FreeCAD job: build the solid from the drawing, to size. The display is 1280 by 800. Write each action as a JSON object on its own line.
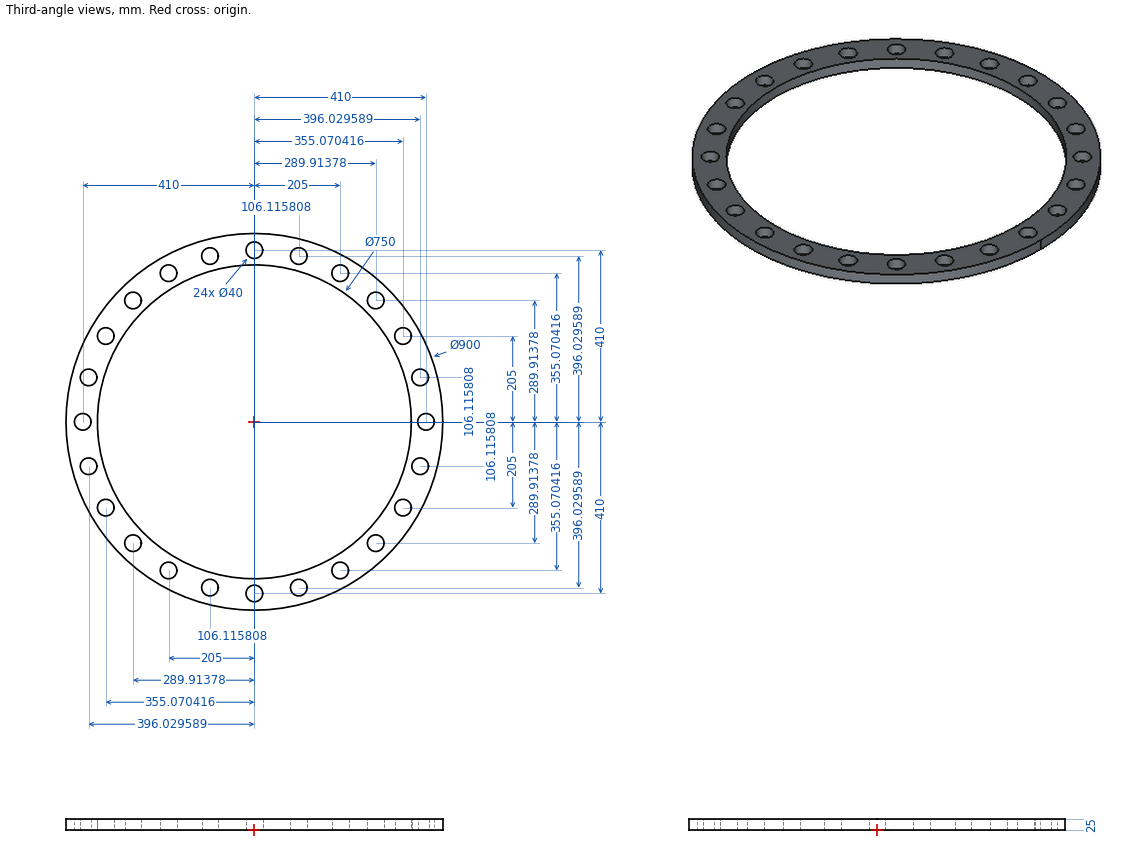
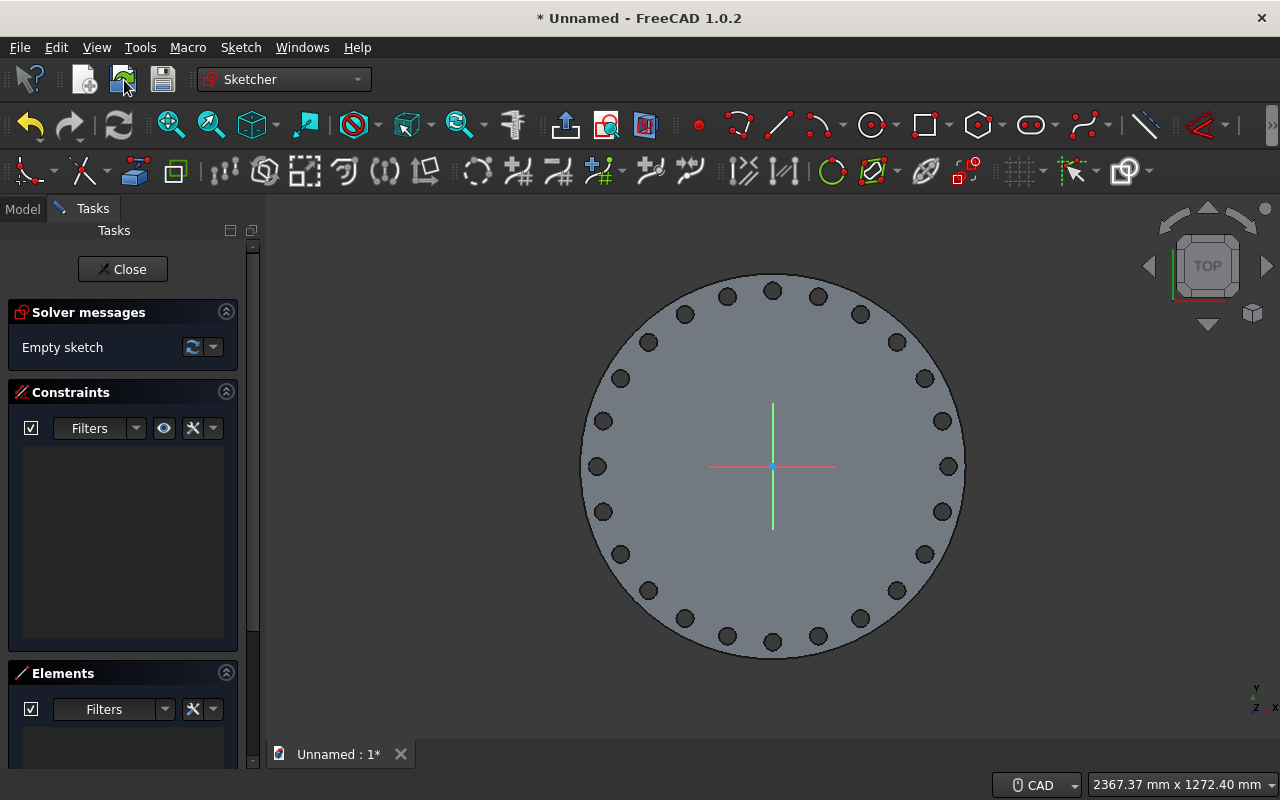
{"action": "left_click", "coordinate": [872, 126]}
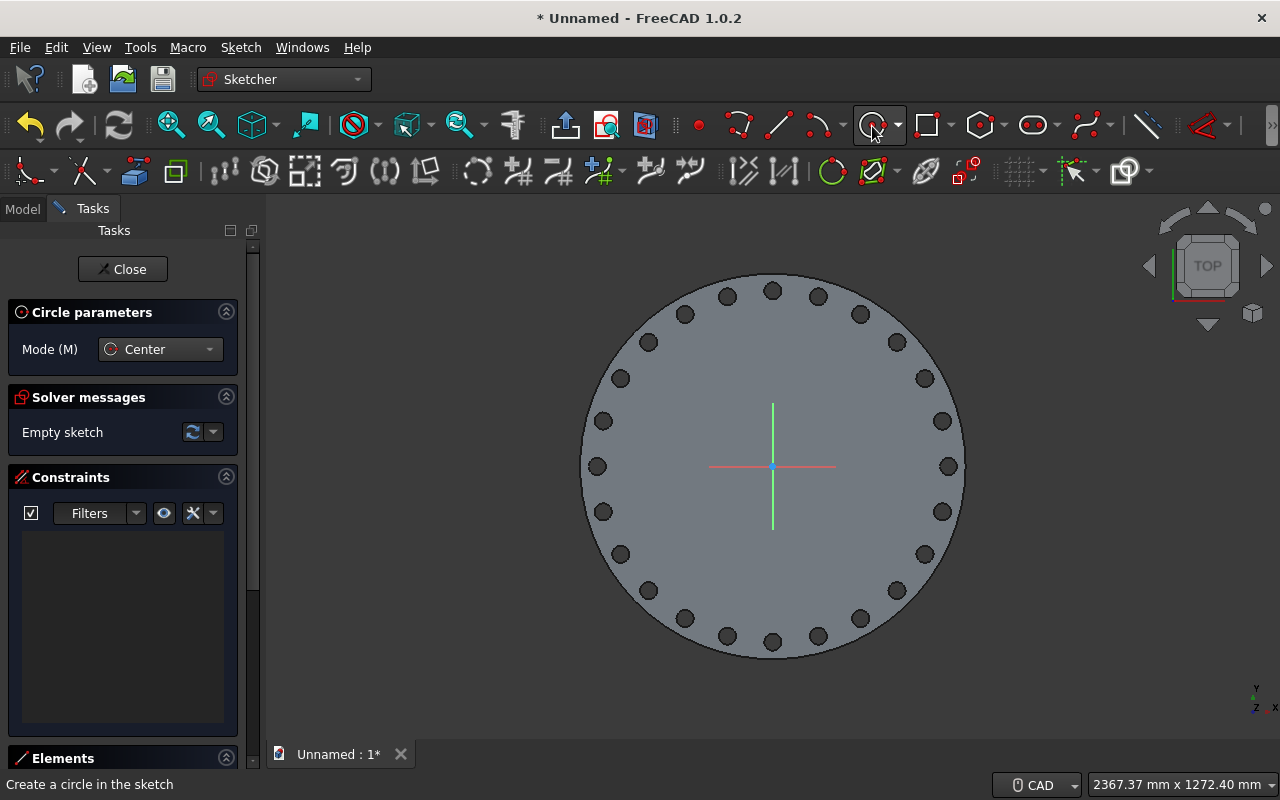
{"action": "left_click", "coordinate": [773, 466]}
{"action": "mouse_move", "coordinate": [886, 353]}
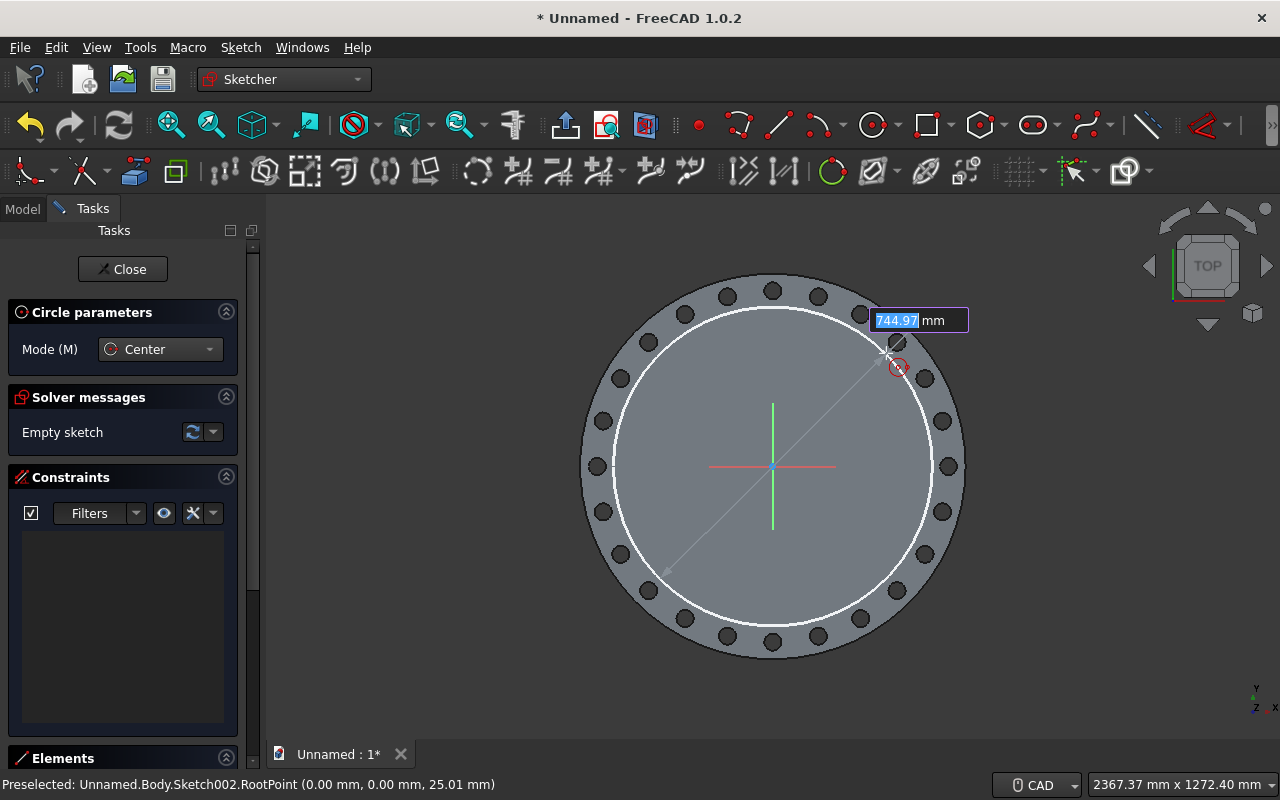
{"action": "type", "text": "750"}
{"action": "key", "text": "Return"}
{"action": "key", "text": "Escape"}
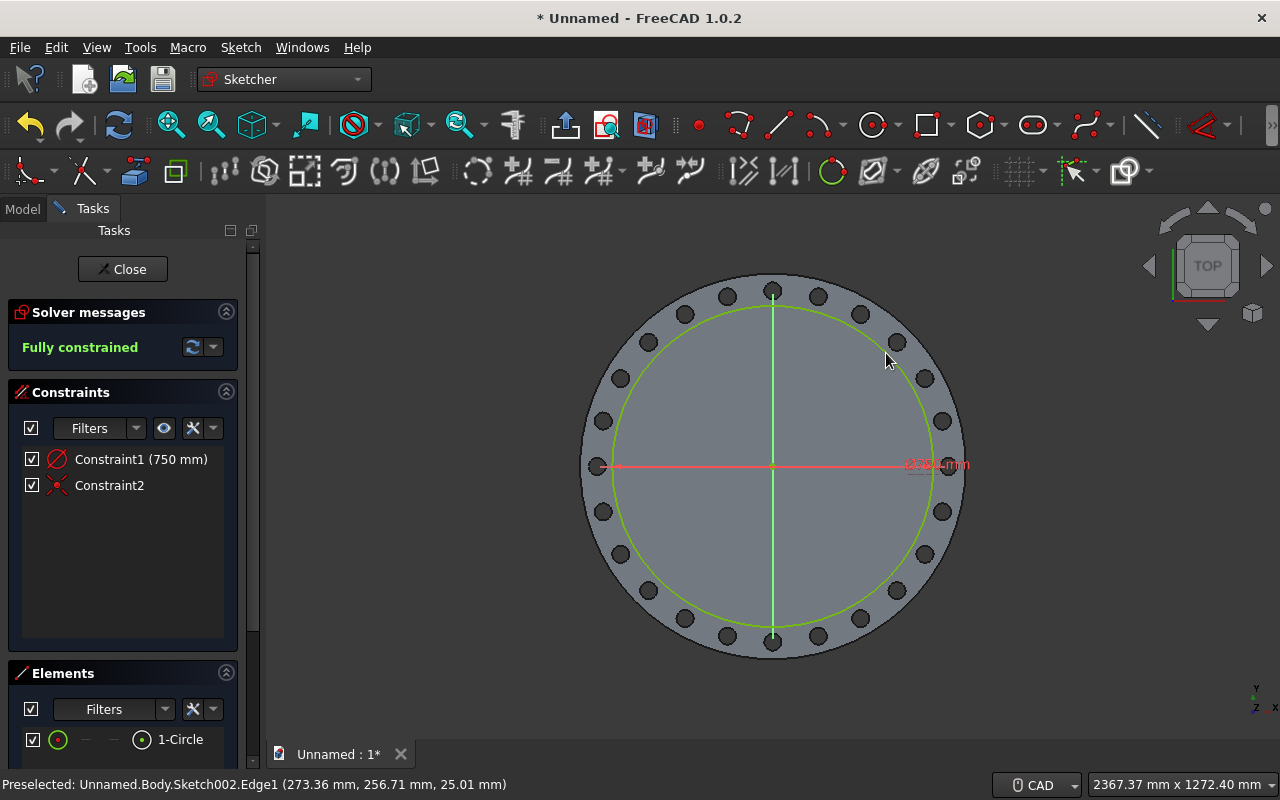
{"action": "left_click", "coordinate": [123, 269]}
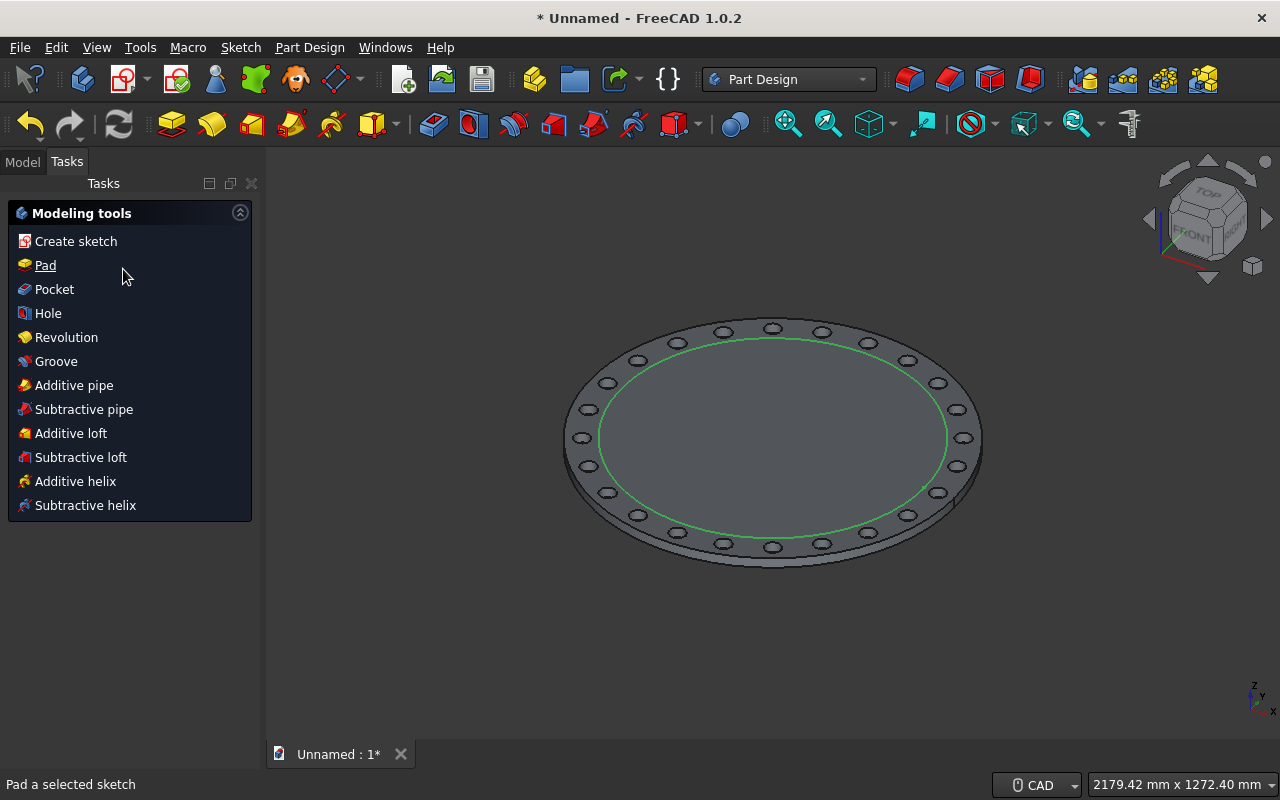
{"action": "left_click", "coordinate": [434, 124]}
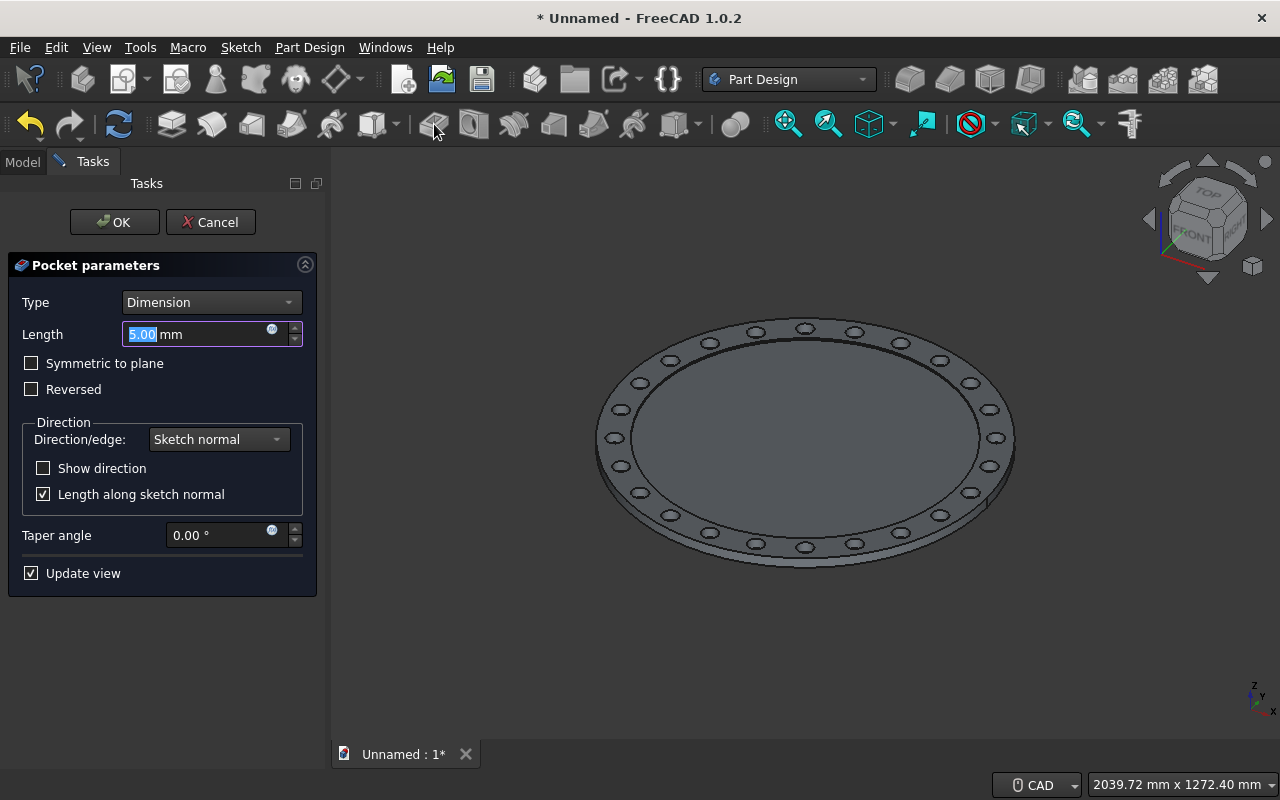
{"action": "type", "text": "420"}
{"action": "key", "text": "Tab"}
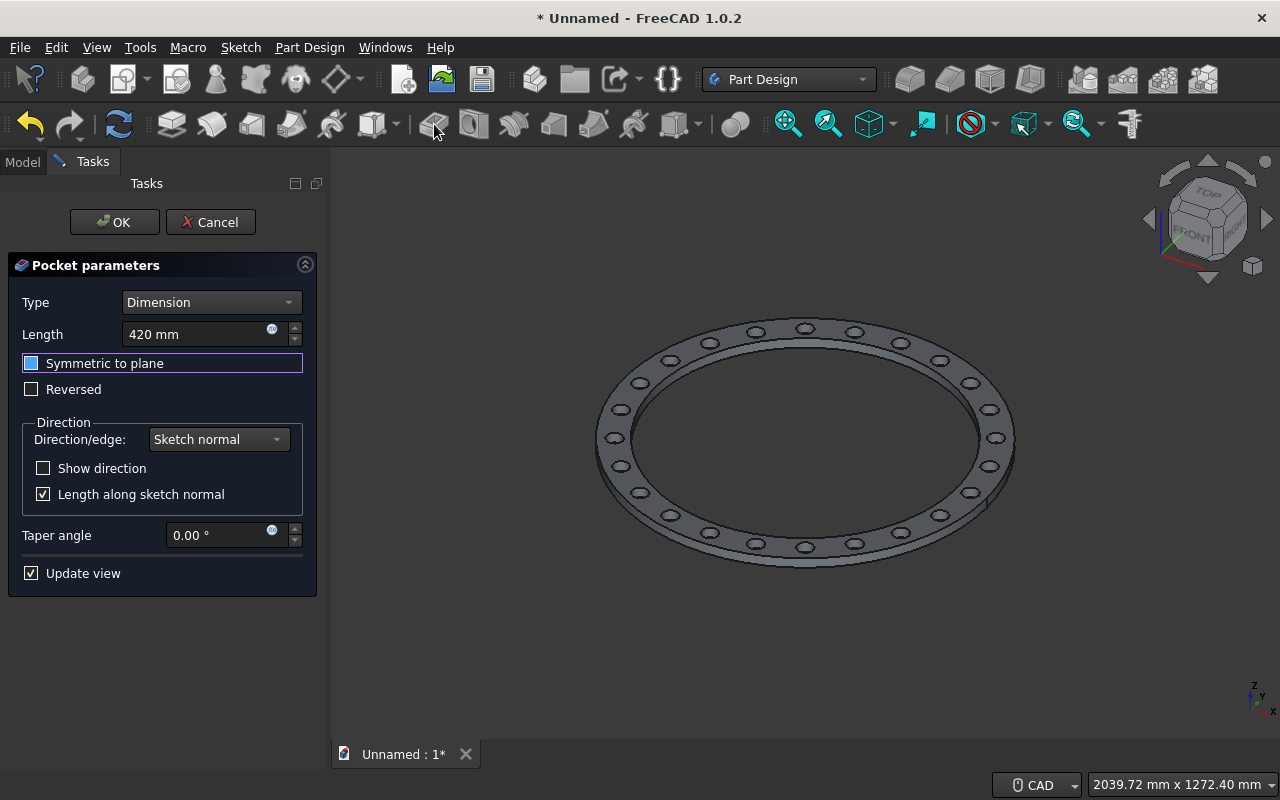
{"action": "left_click", "coordinate": [115, 222]}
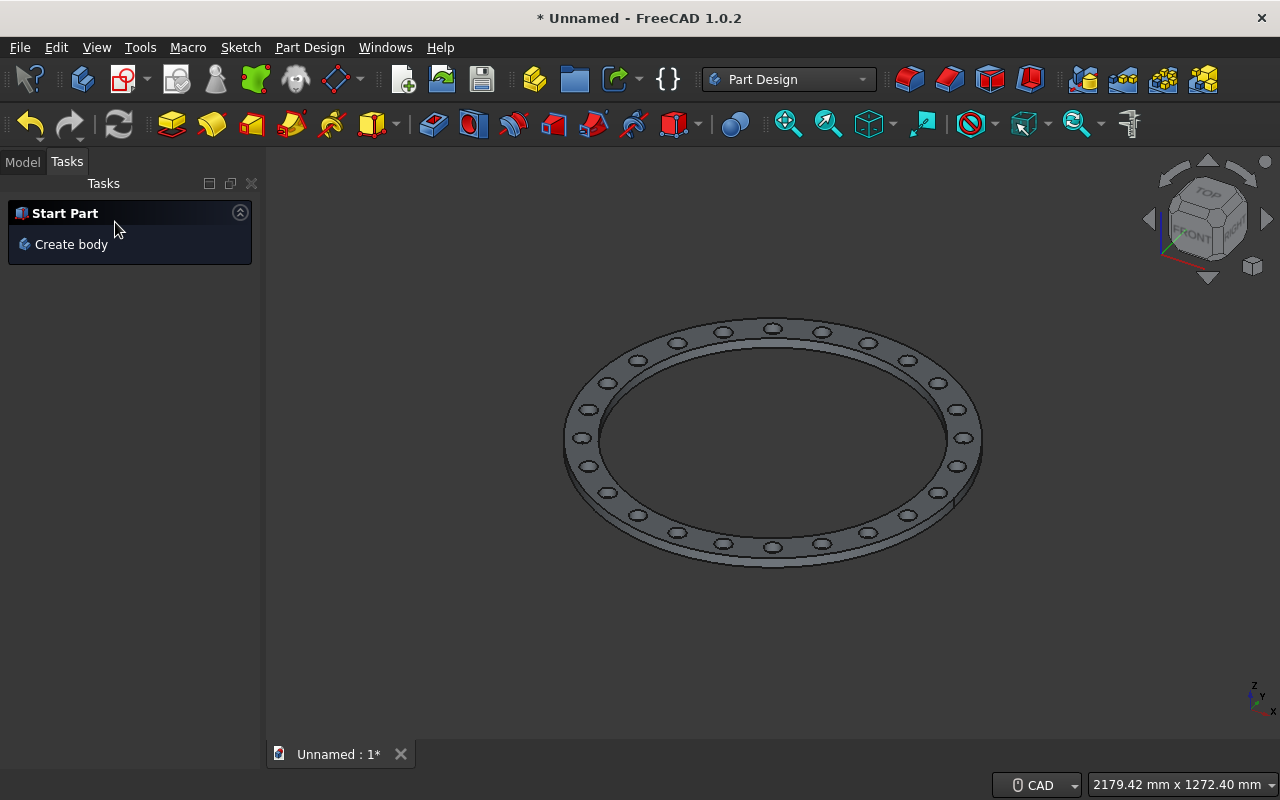
{"action": "key", "text": "0"}